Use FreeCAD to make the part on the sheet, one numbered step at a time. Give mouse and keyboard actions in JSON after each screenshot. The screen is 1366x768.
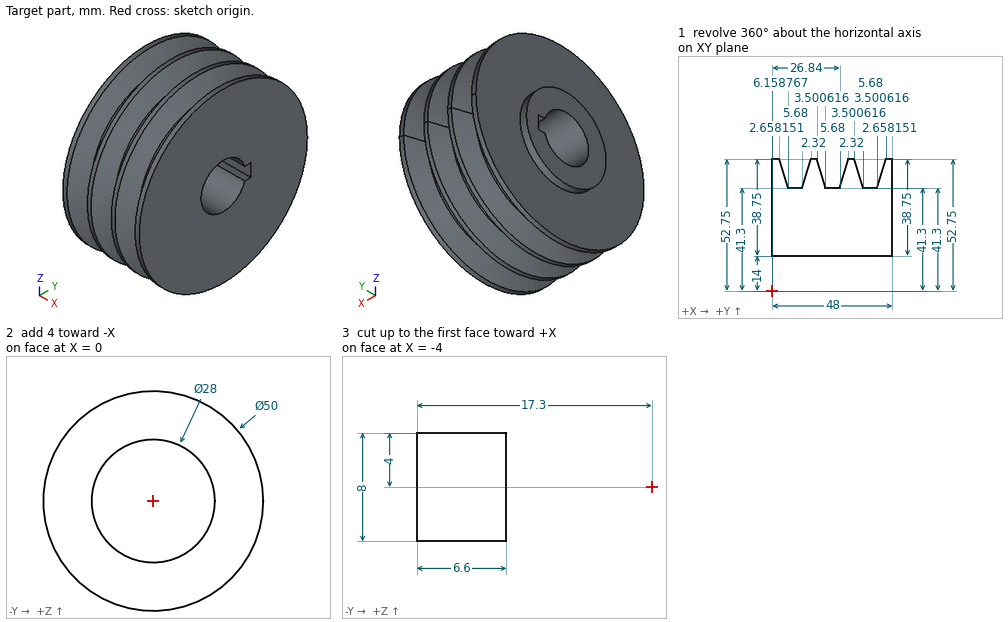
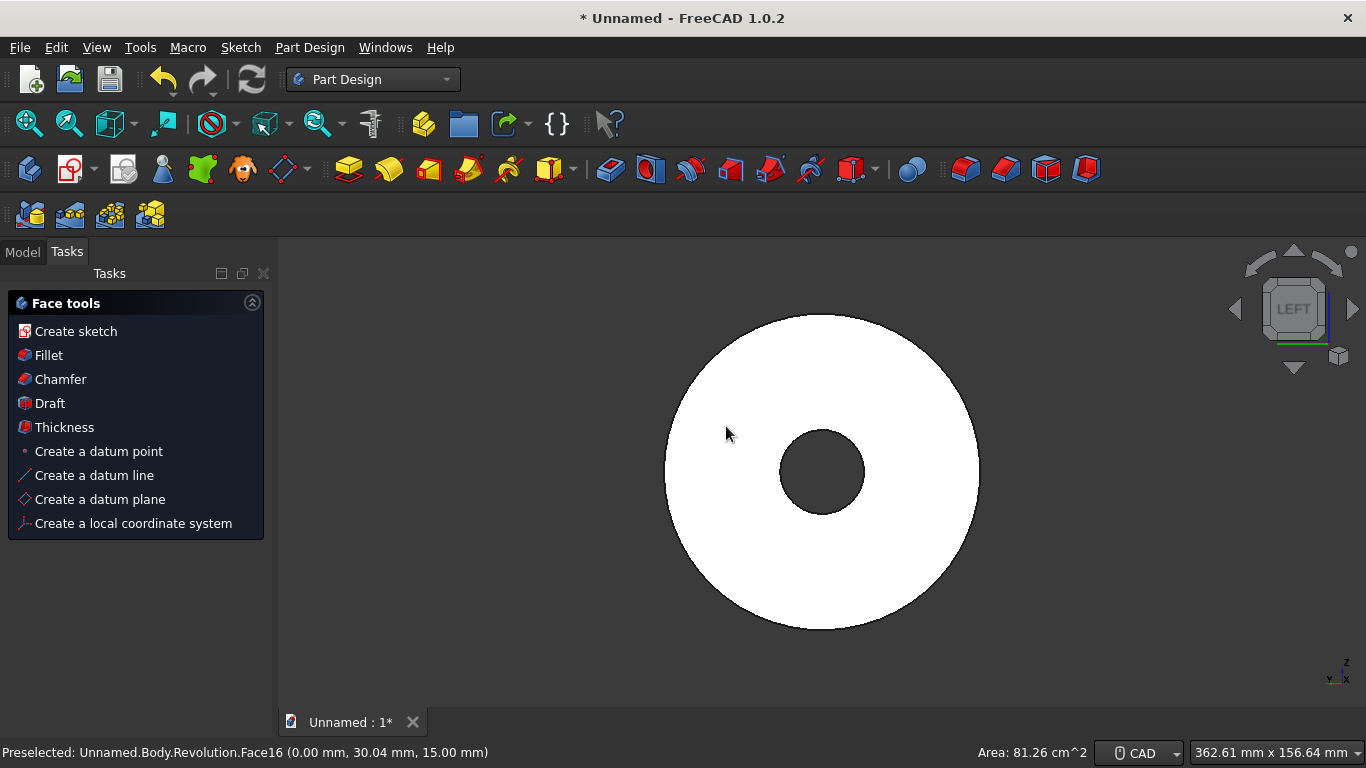
{"action": "left_click", "coordinate": [70, 170]}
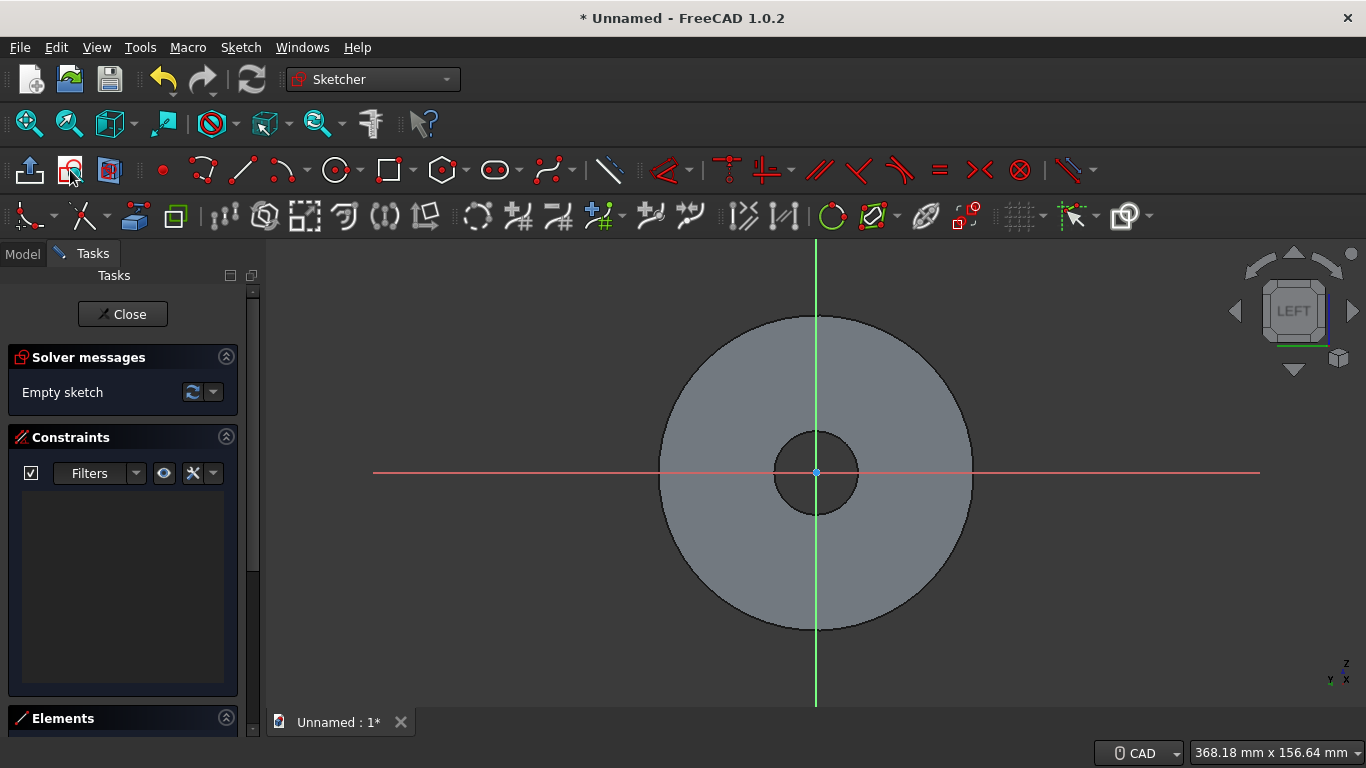
{"action": "scroll", "coordinate": [900, 473], "scroll_direction": "up", "scroll_amount": 3}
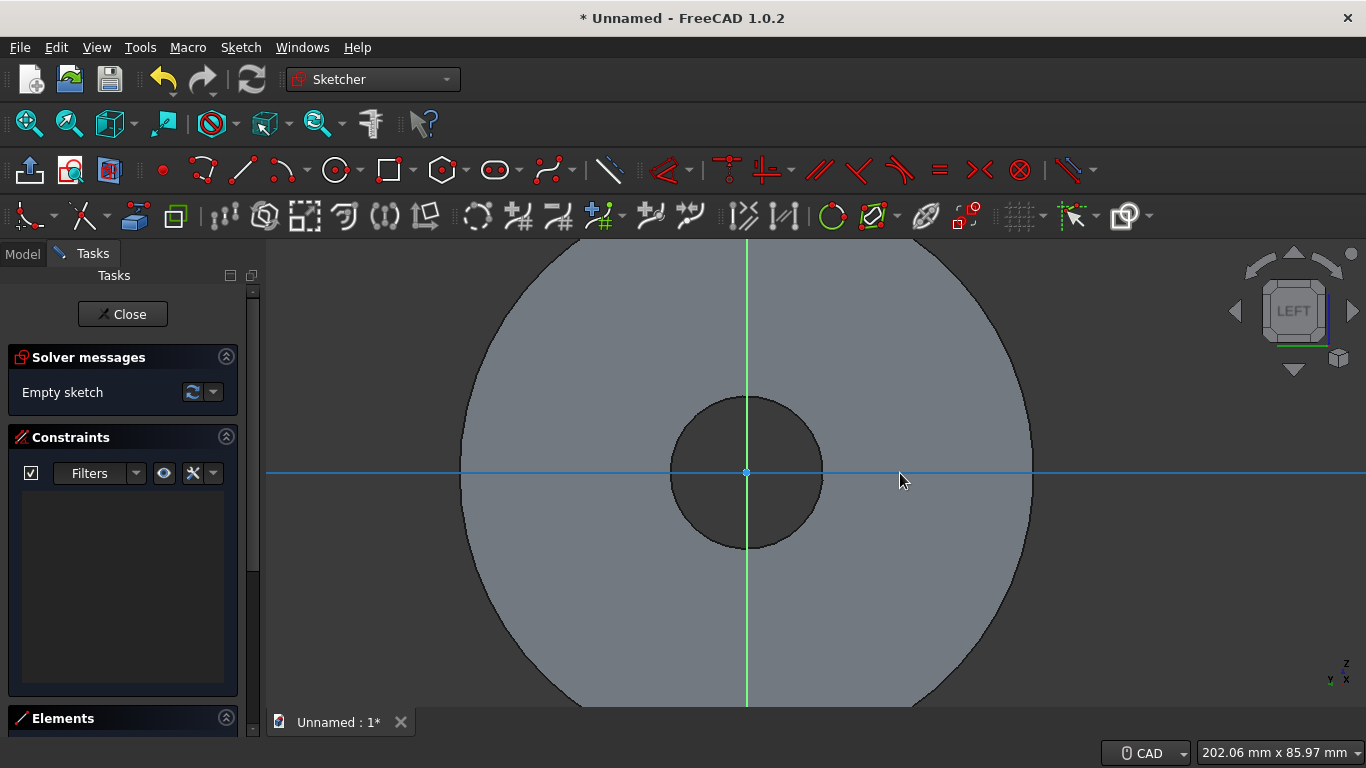
{"action": "left_click", "coordinate": [336, 170]}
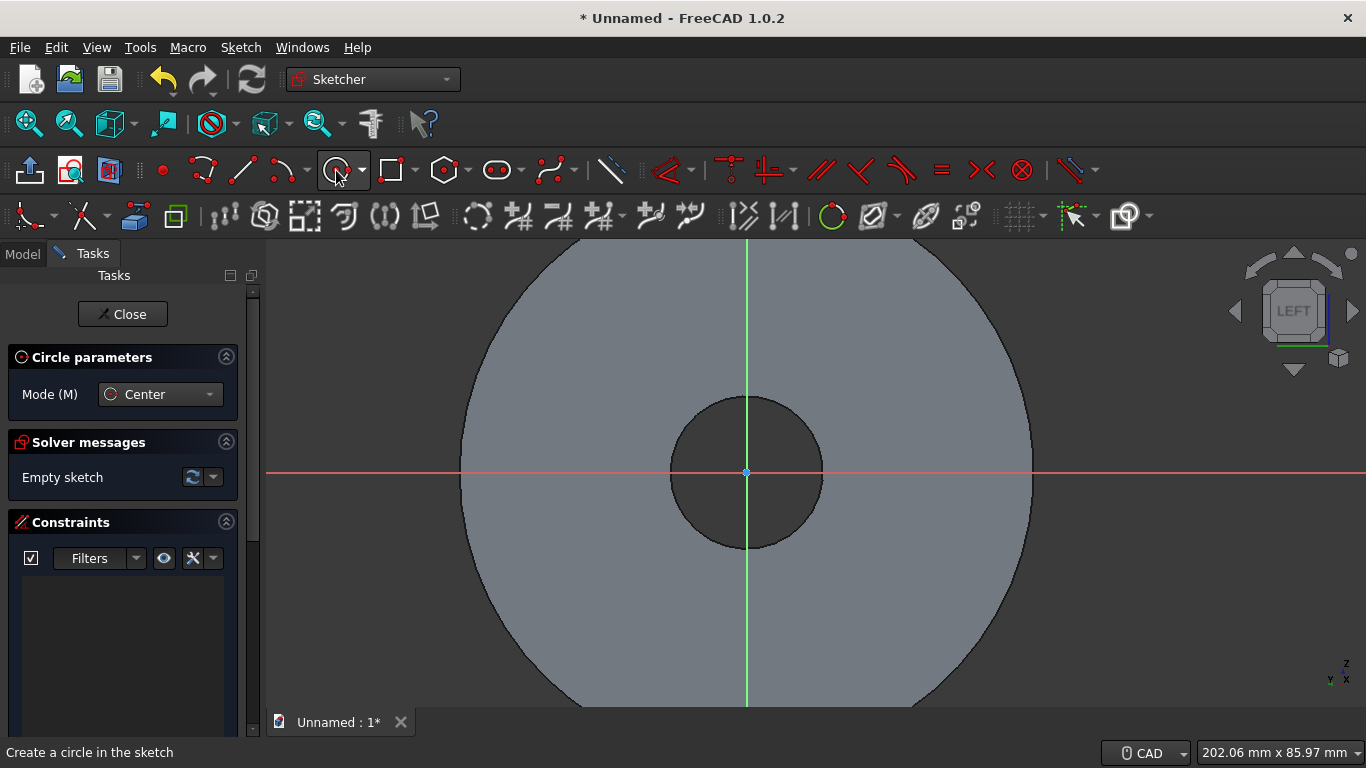
{"action": "left_click", "coordinate": [747, 473]}
{"action": "left_click", "coordinate": [843, 376]}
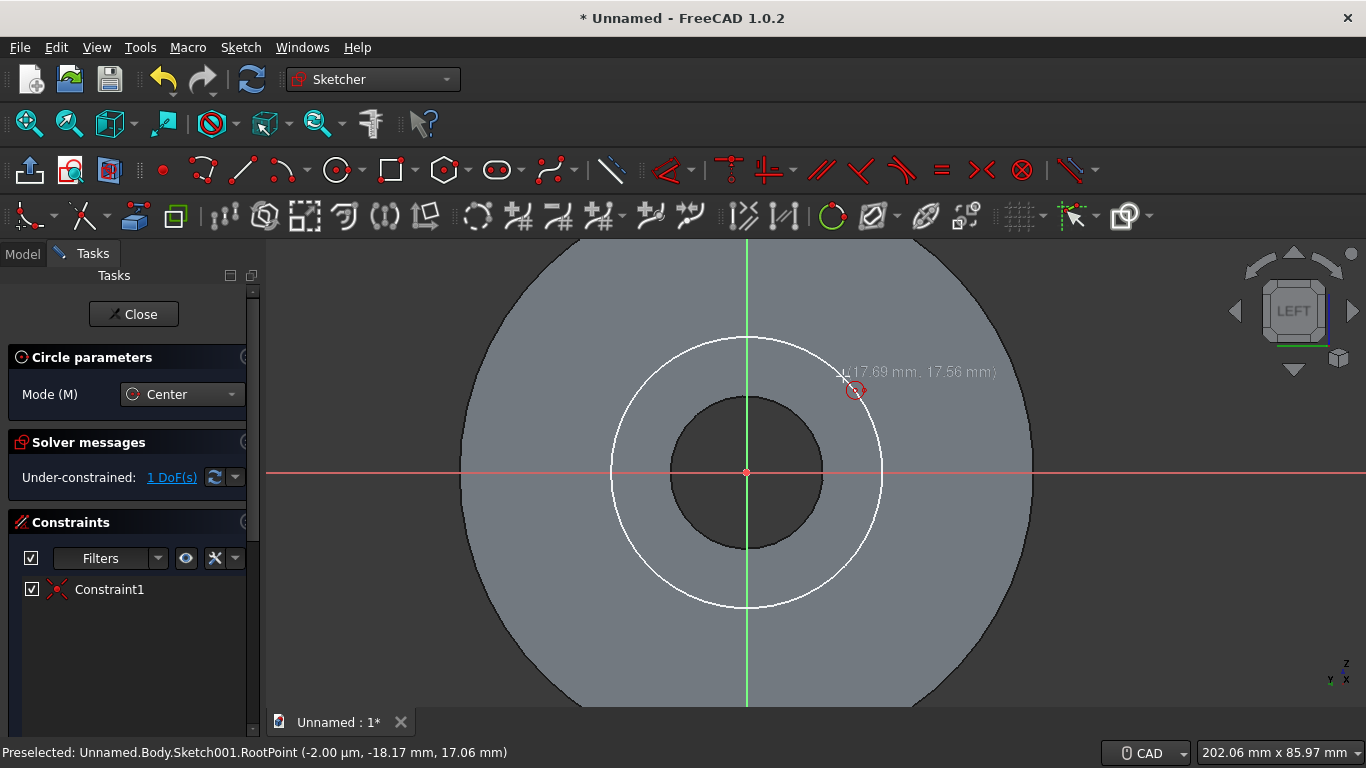
{"action": "left_click", "coordinate": [747, 473]}
{"action": "left_click", "coordinate": [801, 419]}
{"action": "key", "text": "Escape"}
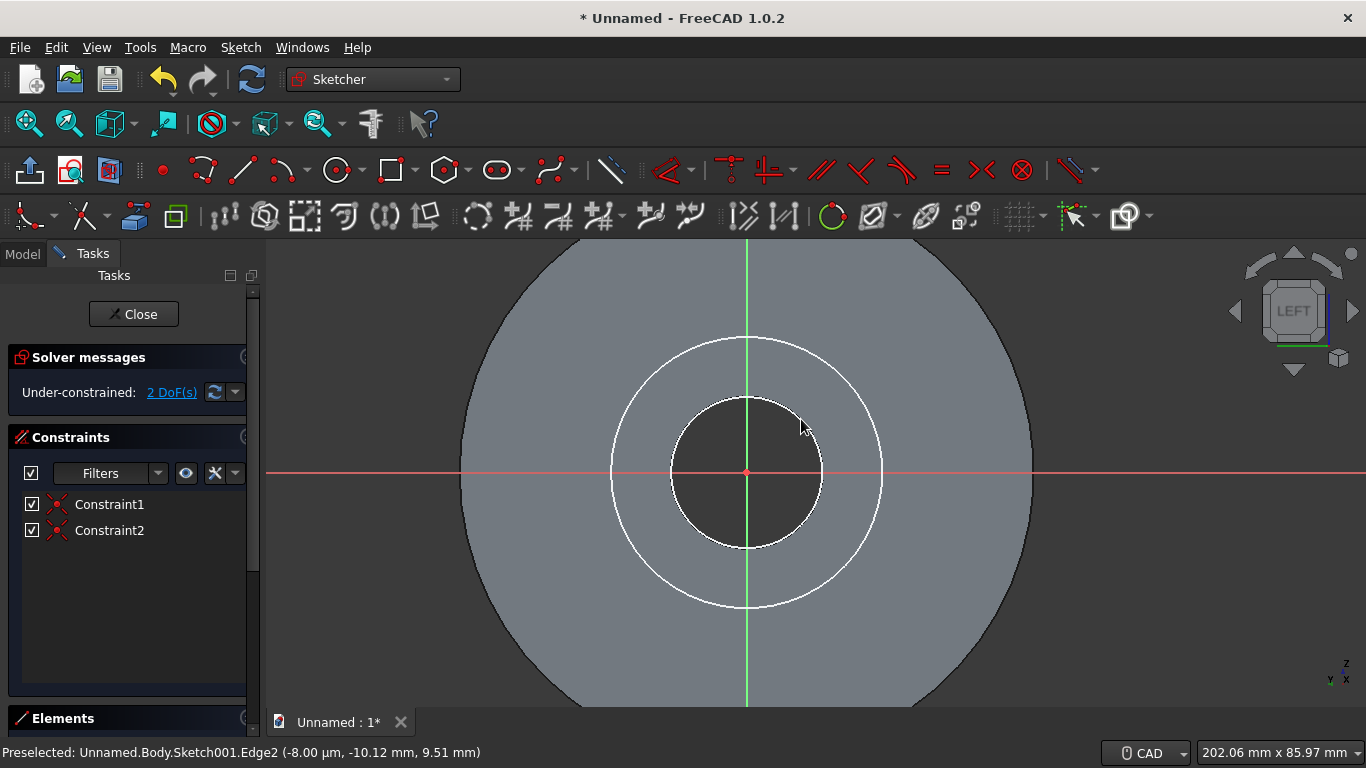
{"action": "left_click", "coordinate": [666, 170]}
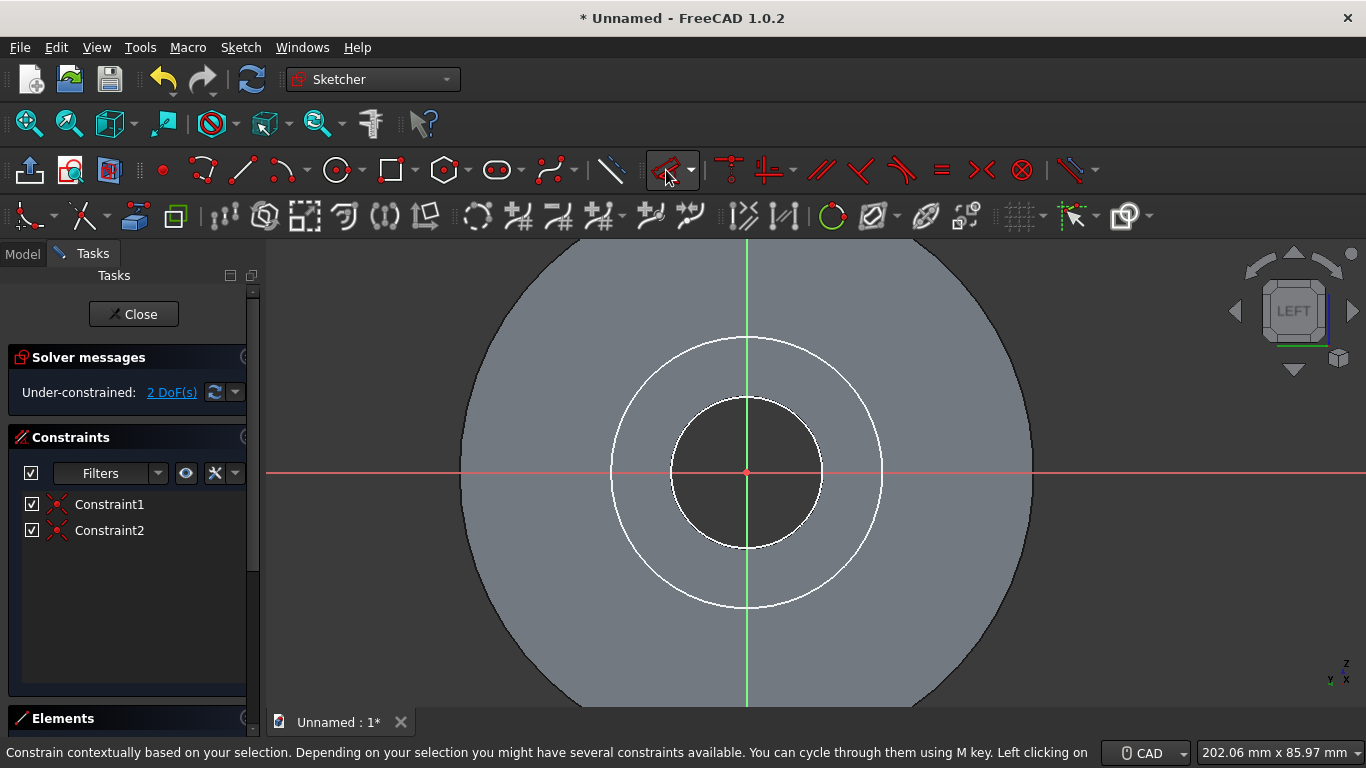
{"action": "left_click", "coordinate": [842, 376]}
{"action": "left_click", "coordinate": [864, 353]}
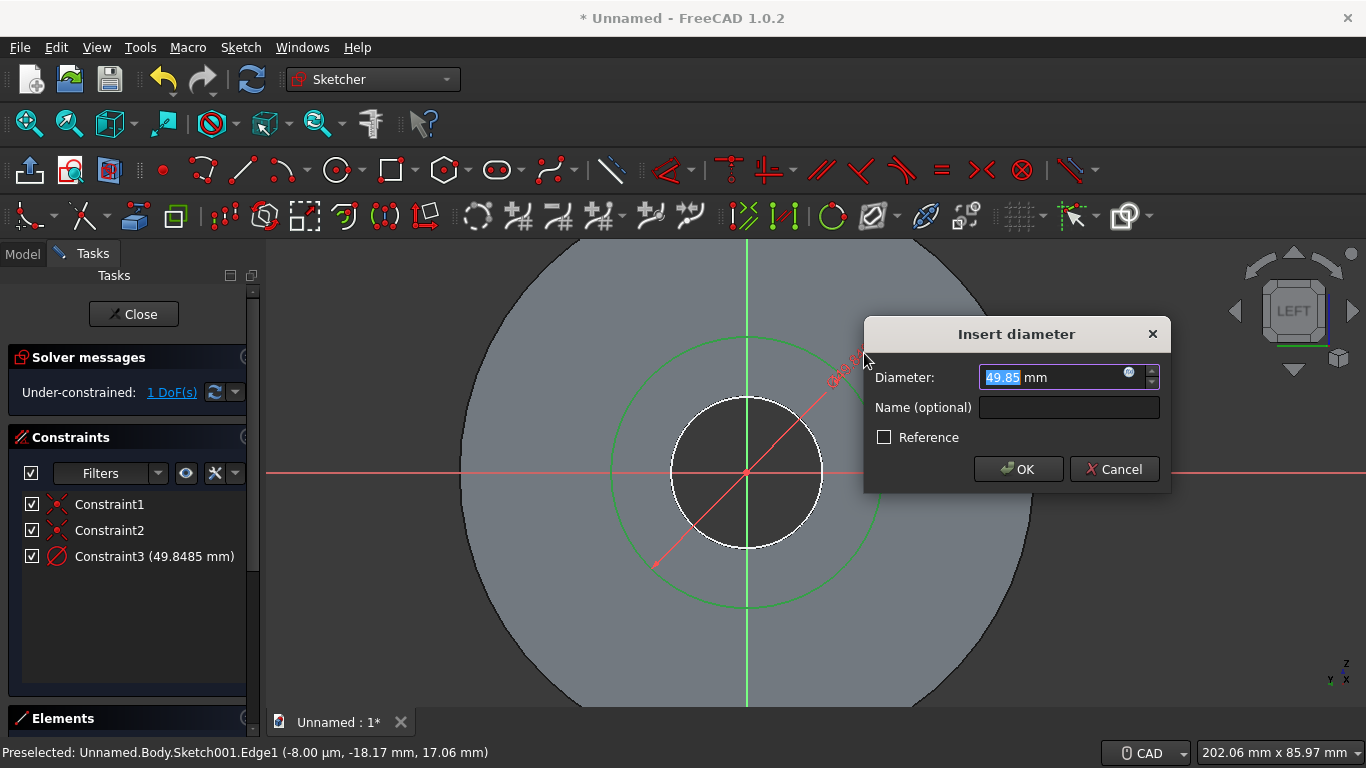
{"action": "type", "text": "50"}
{"action": "key", "text": "Return"}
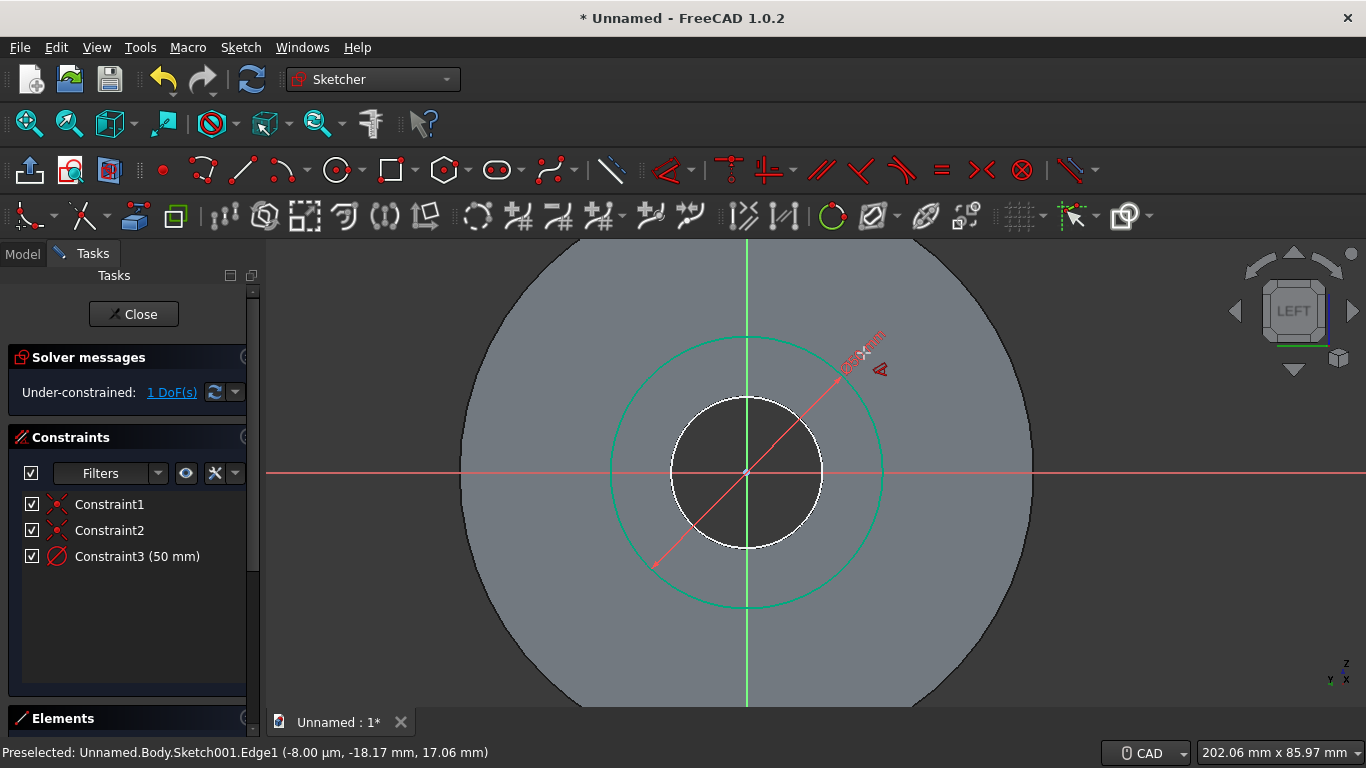
{"action": "left_click", "coordinate": [800, 419]}
{"action": "left_click", "coordinate": [823, 396]}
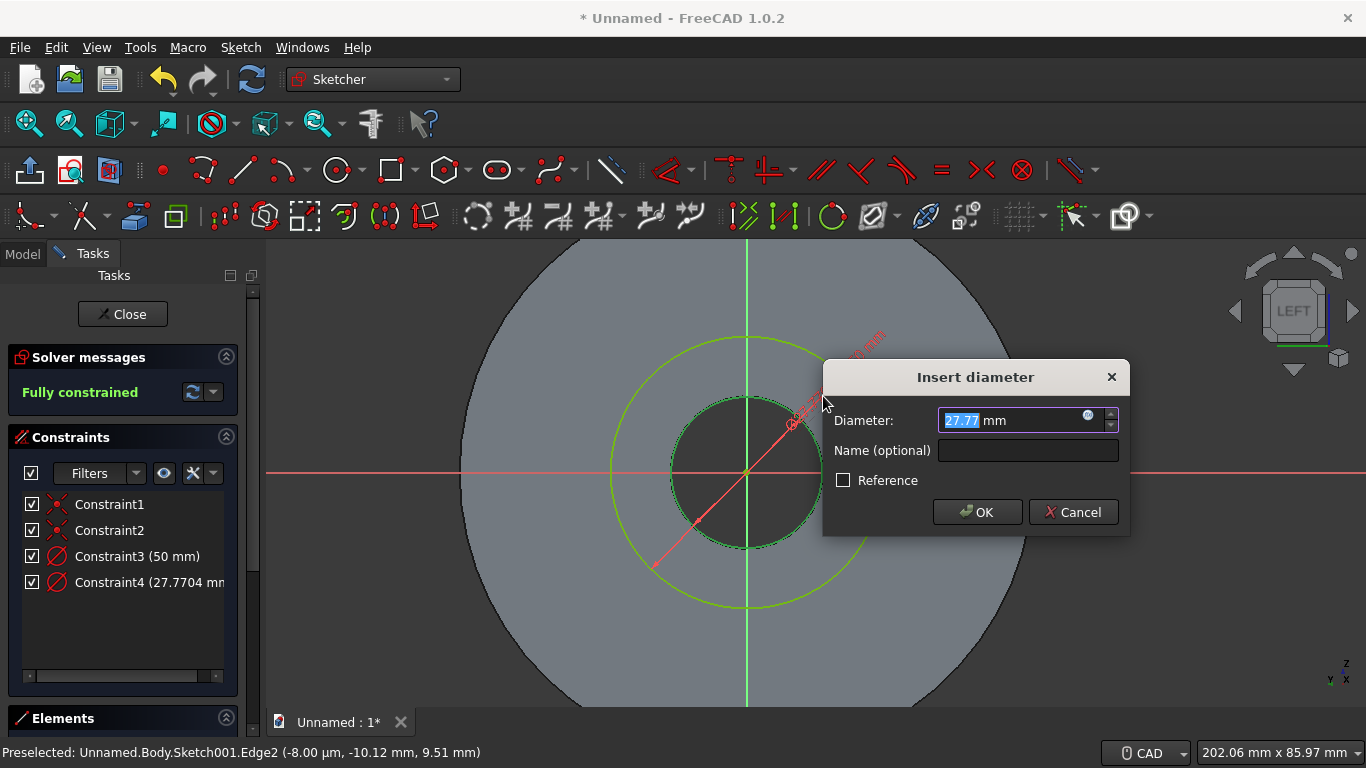
{"action": "type", "text": "28"}
{"action": "key", "text": "Return"}
{"action": "key", "text": "Escape"}